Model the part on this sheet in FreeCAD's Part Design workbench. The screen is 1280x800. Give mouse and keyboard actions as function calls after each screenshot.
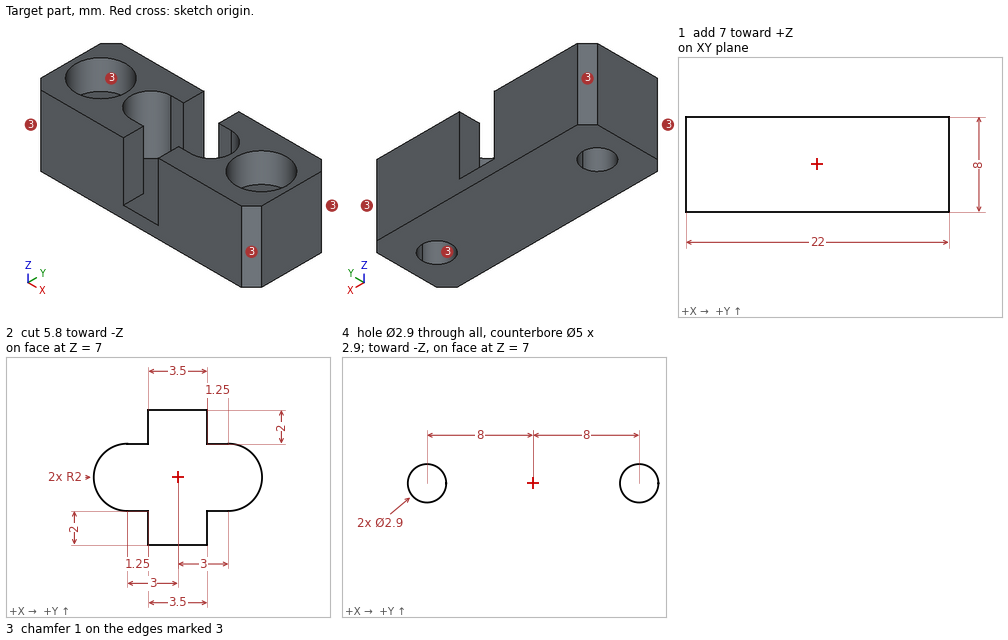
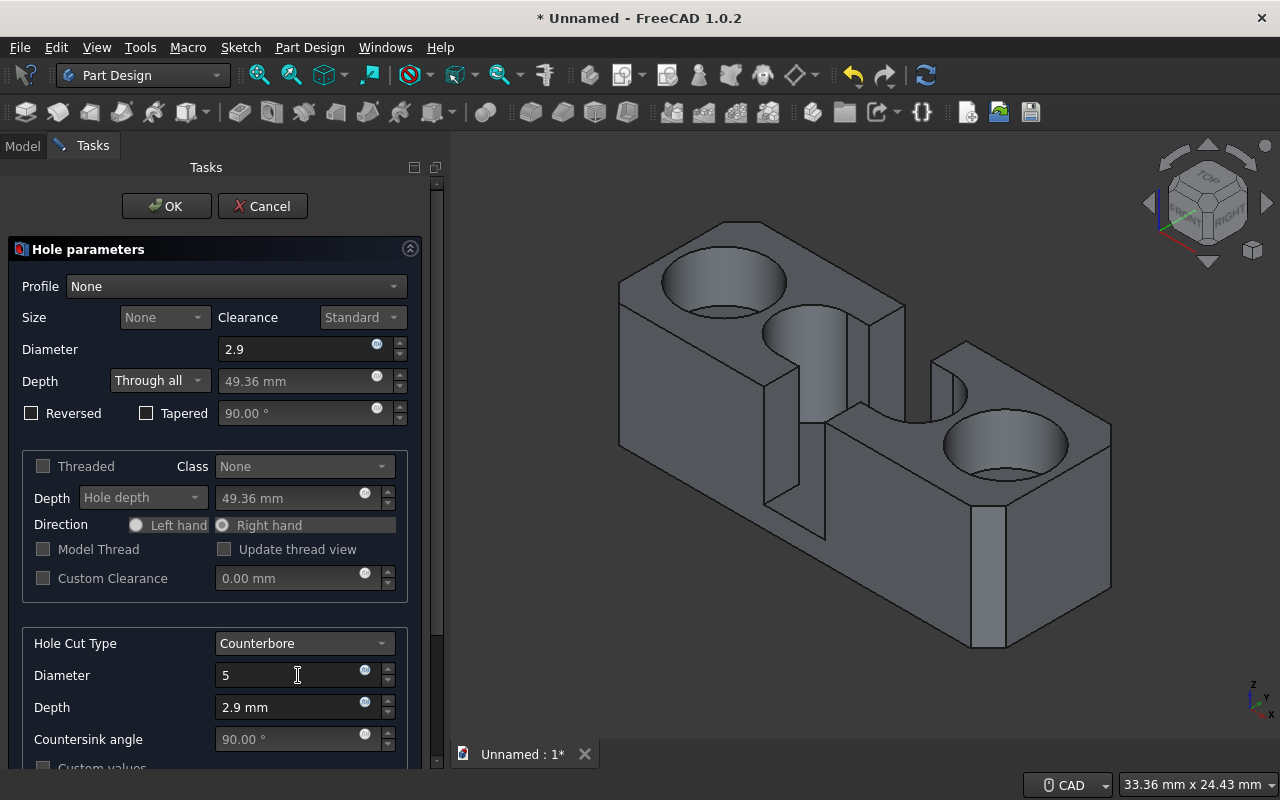
click(167, 206)